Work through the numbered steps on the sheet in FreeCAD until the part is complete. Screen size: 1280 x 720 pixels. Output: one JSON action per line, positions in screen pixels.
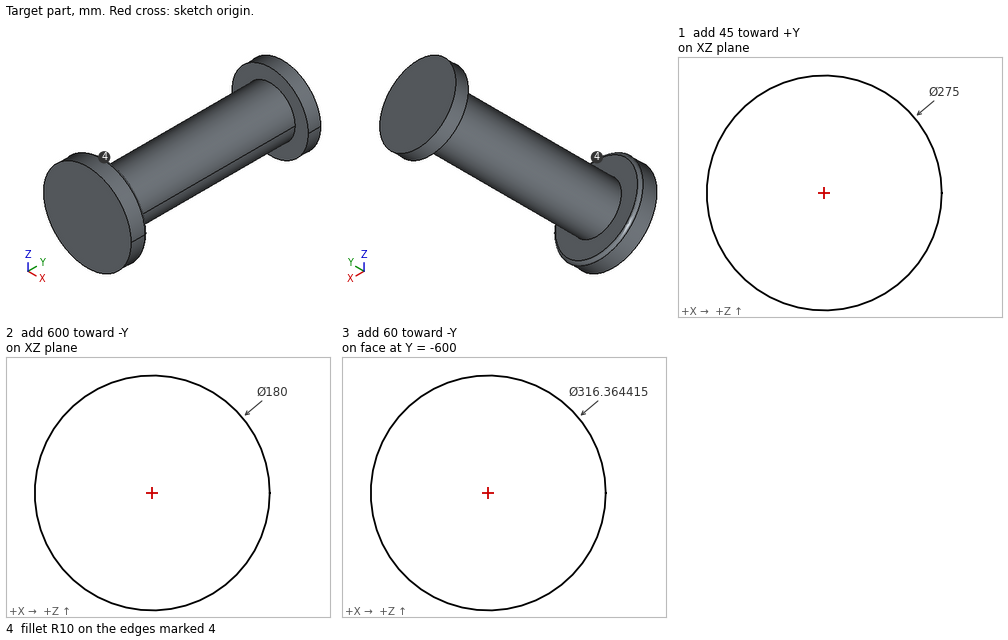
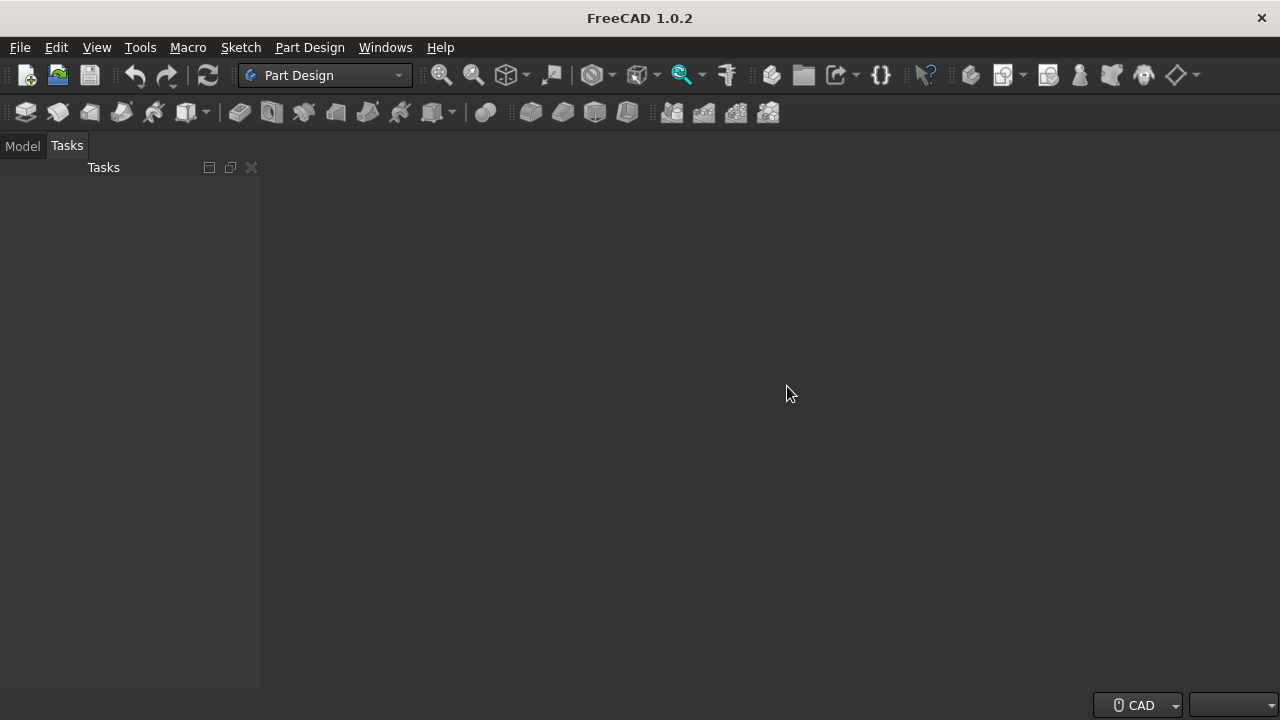
{"action": "key", "text": "ctrl+n"}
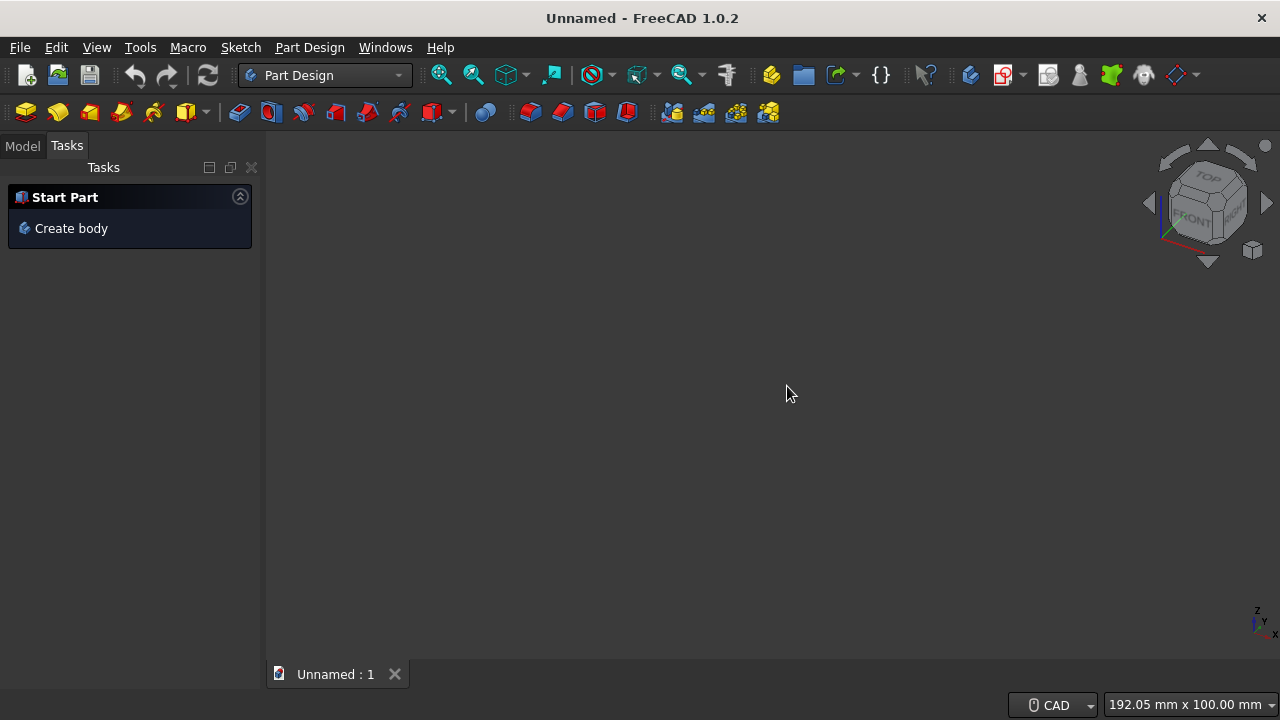
{"action": "left_click", "coordinate": [1004, 76]}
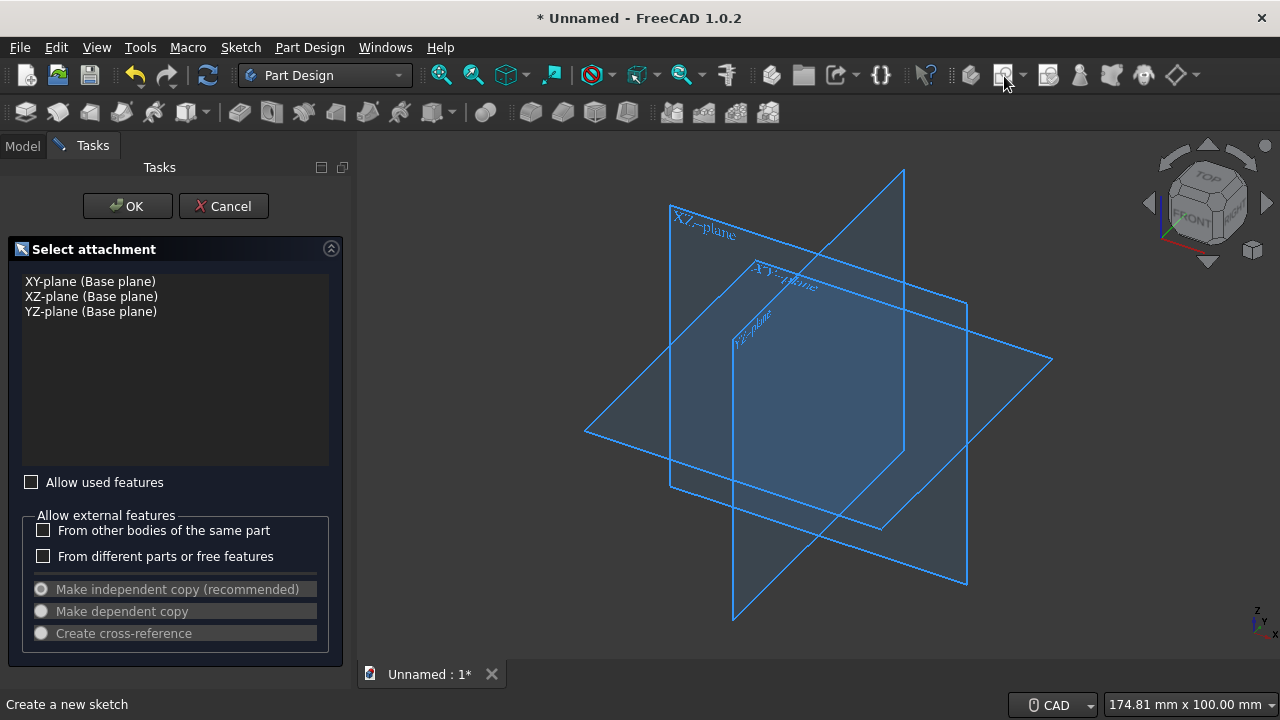
{"action": "left_click", "coordinate": [82, 296]}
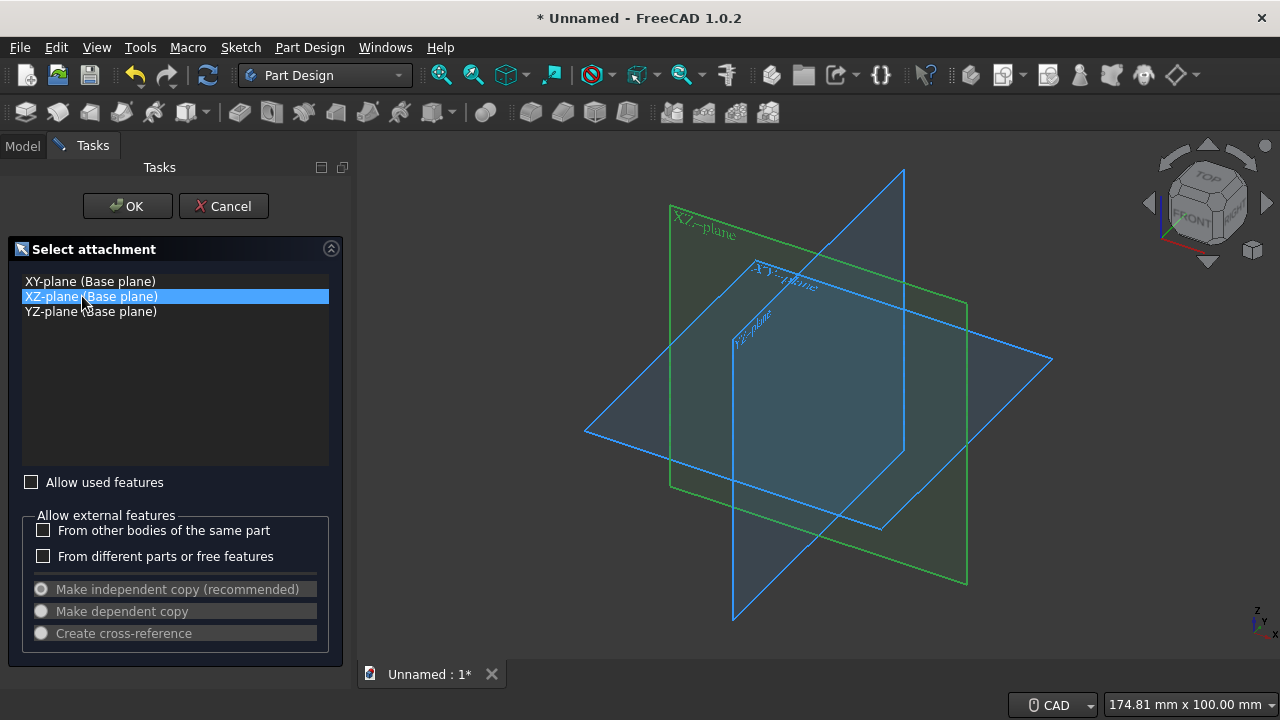
{"action": "left_click", "coordinate": [128, 206]}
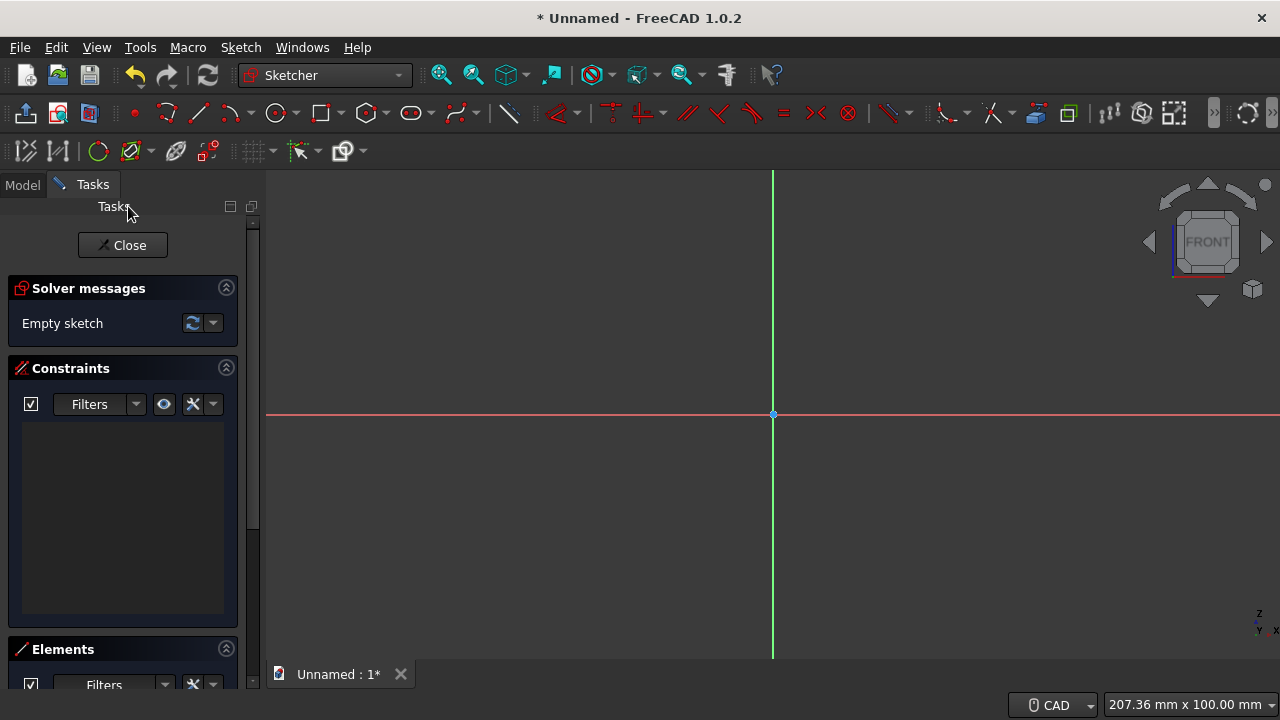
{"action": "scroll", "coordinate": [682, 414], "scroll_direction": "down", "scroll_amount": 7}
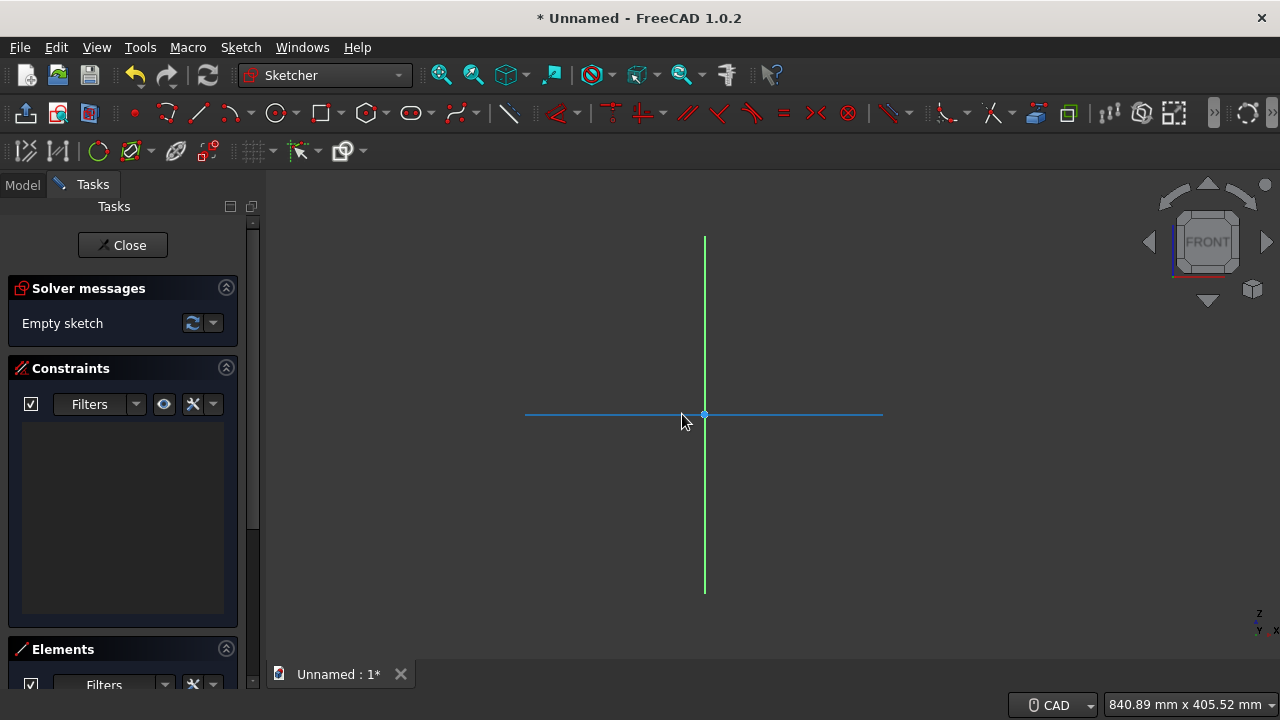
{"action": "key", "text": "g c"}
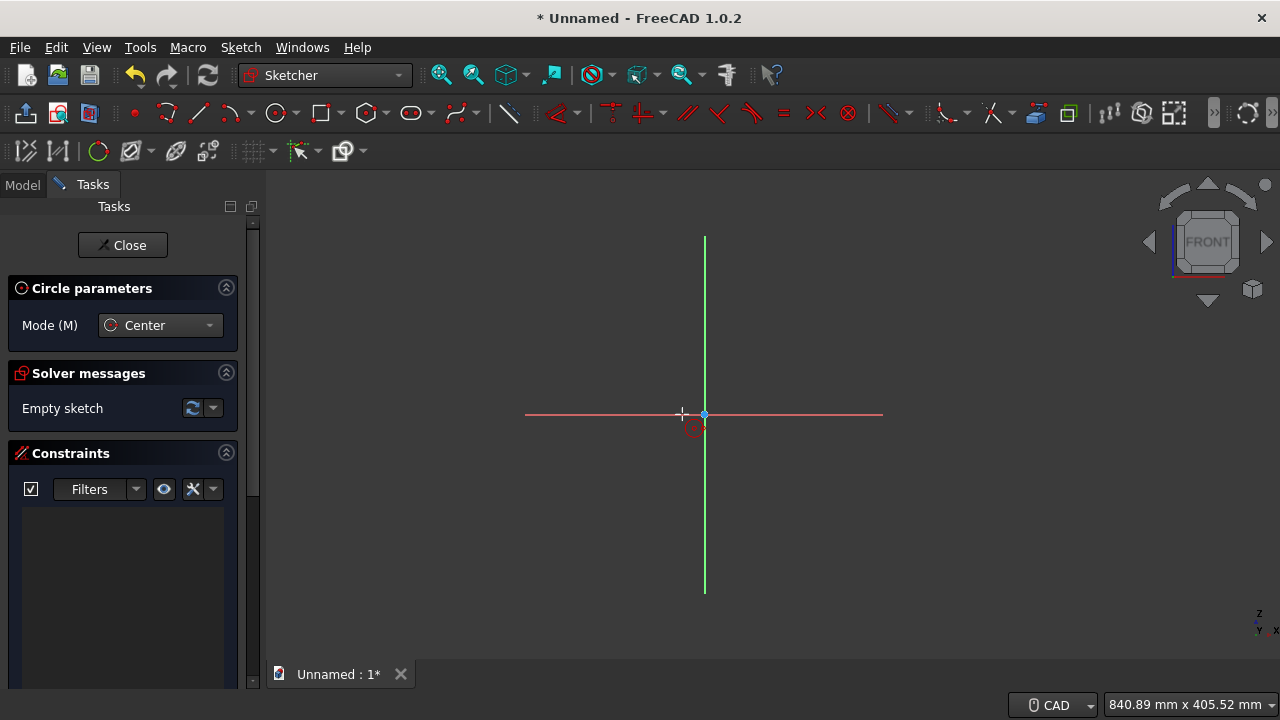
{"action": "left_click", "coordinate": [705, 414]}
{"action": "mouse_move", "coordinate": [822, 297]}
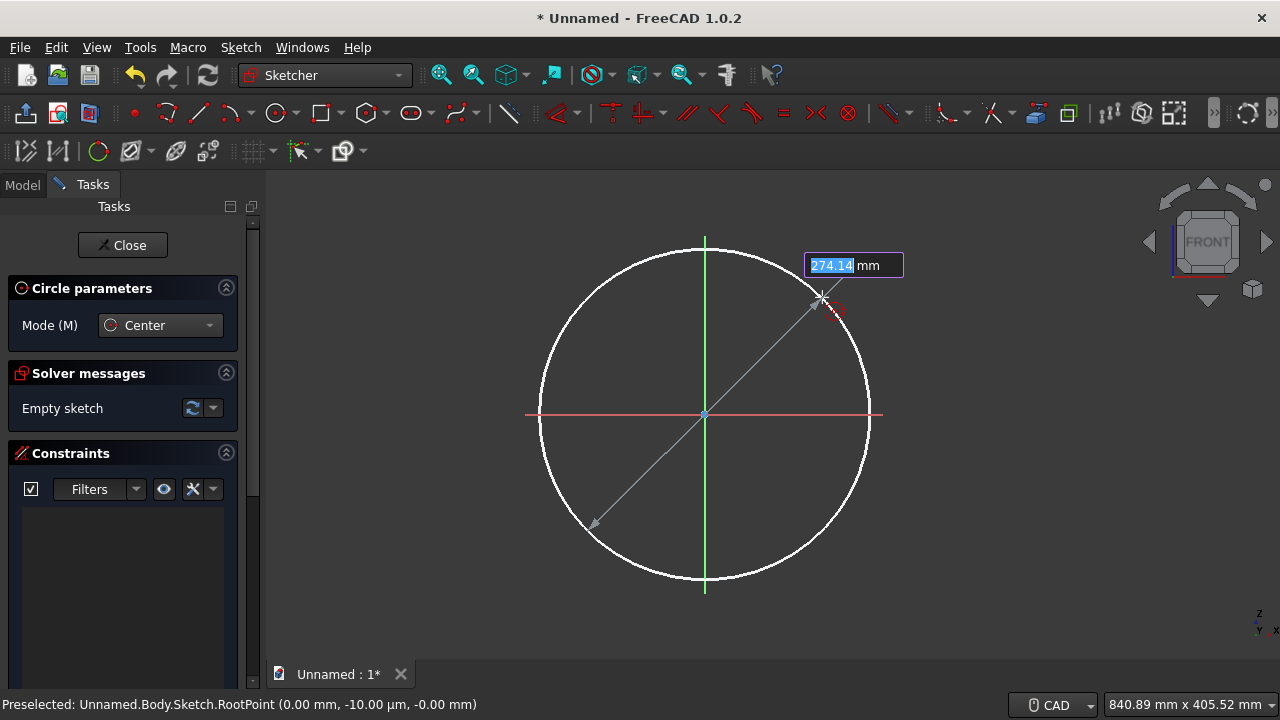
{"action": "type", "text": "275"}
{"action": "key", "text": "Return"}
{"action": "key", "text": "Escape"}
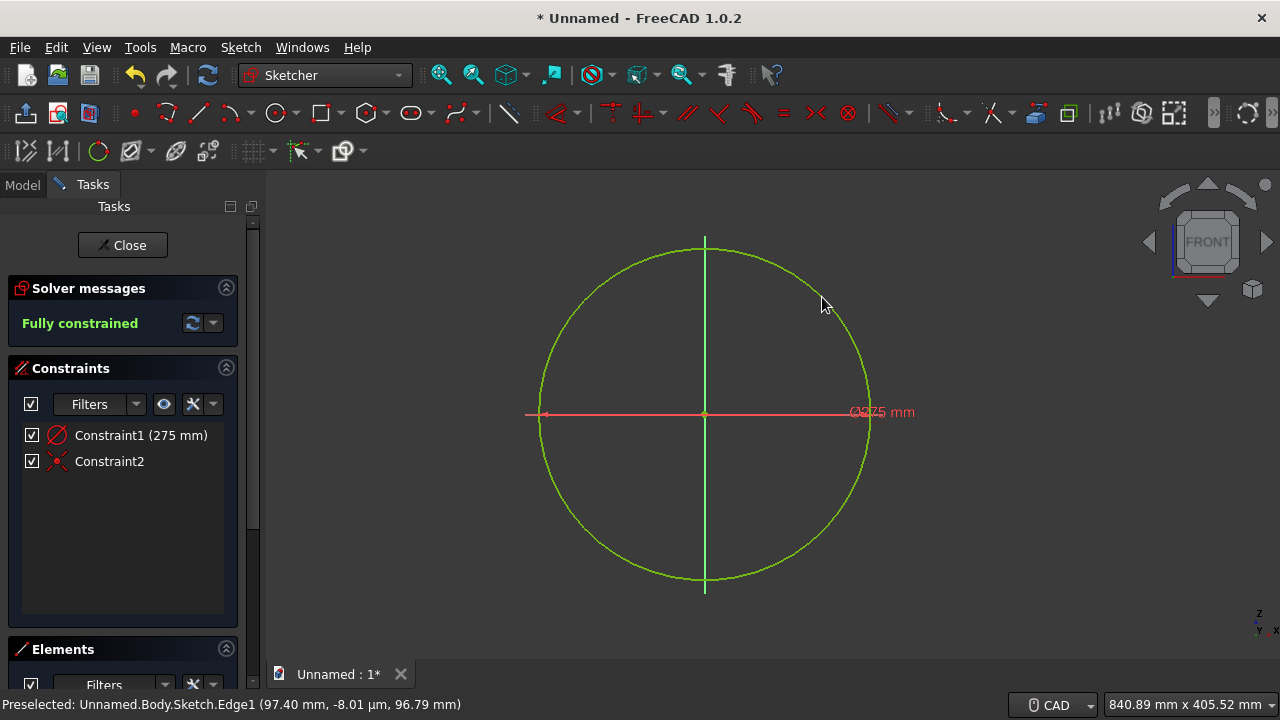
{"action": "left_click", "coordinate": [123, 245]}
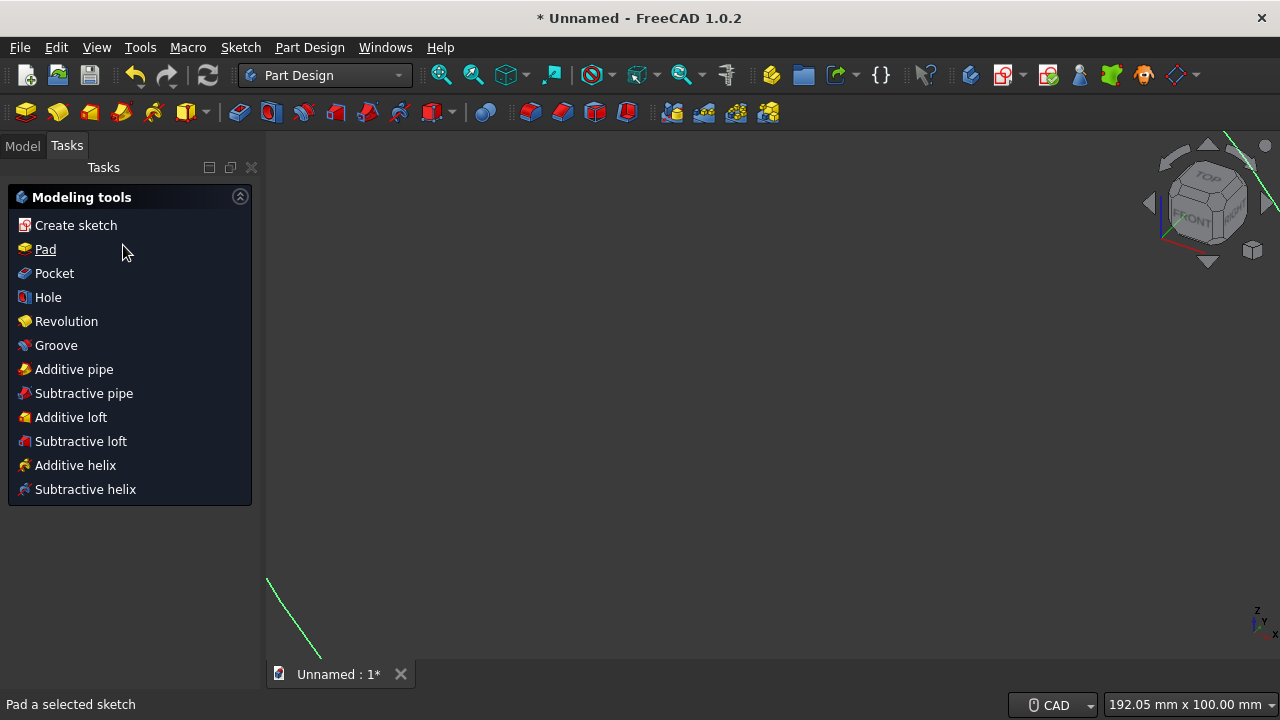
{"action": "left_click", "coordinate": [26, 112]}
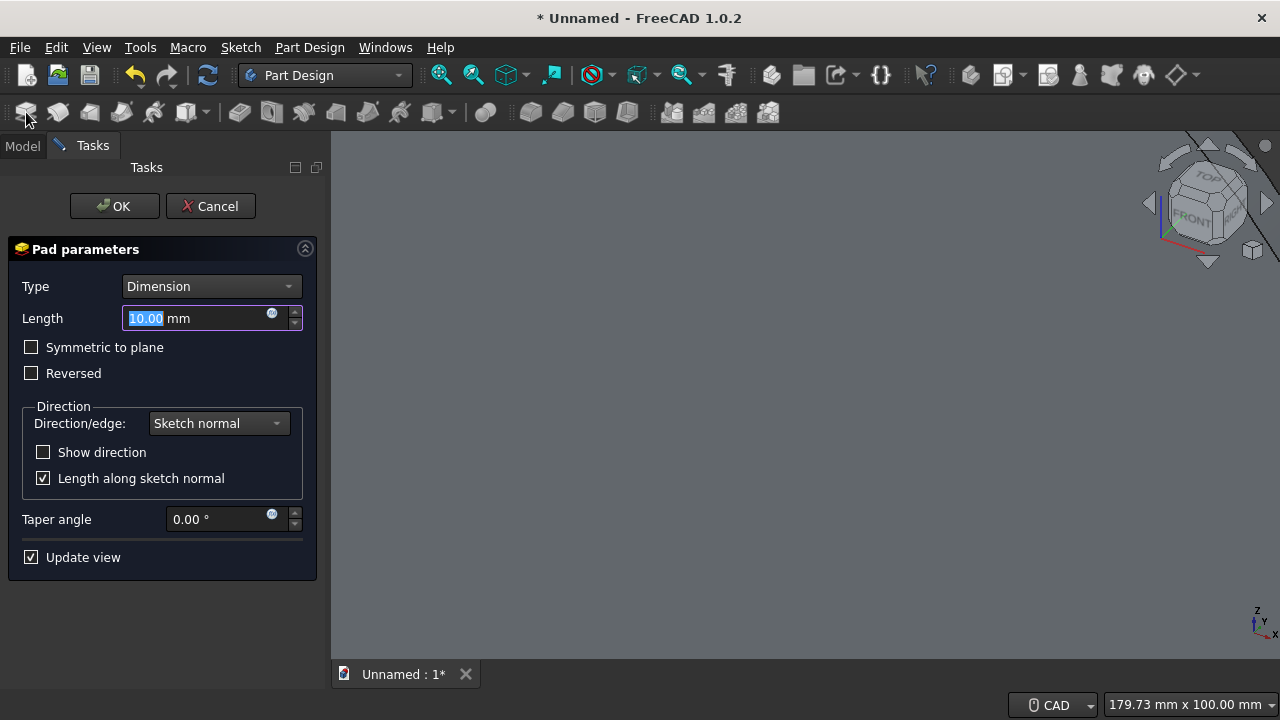
{"action": "type", "text": "45"}
{"action": "key", "text": "Tab"}